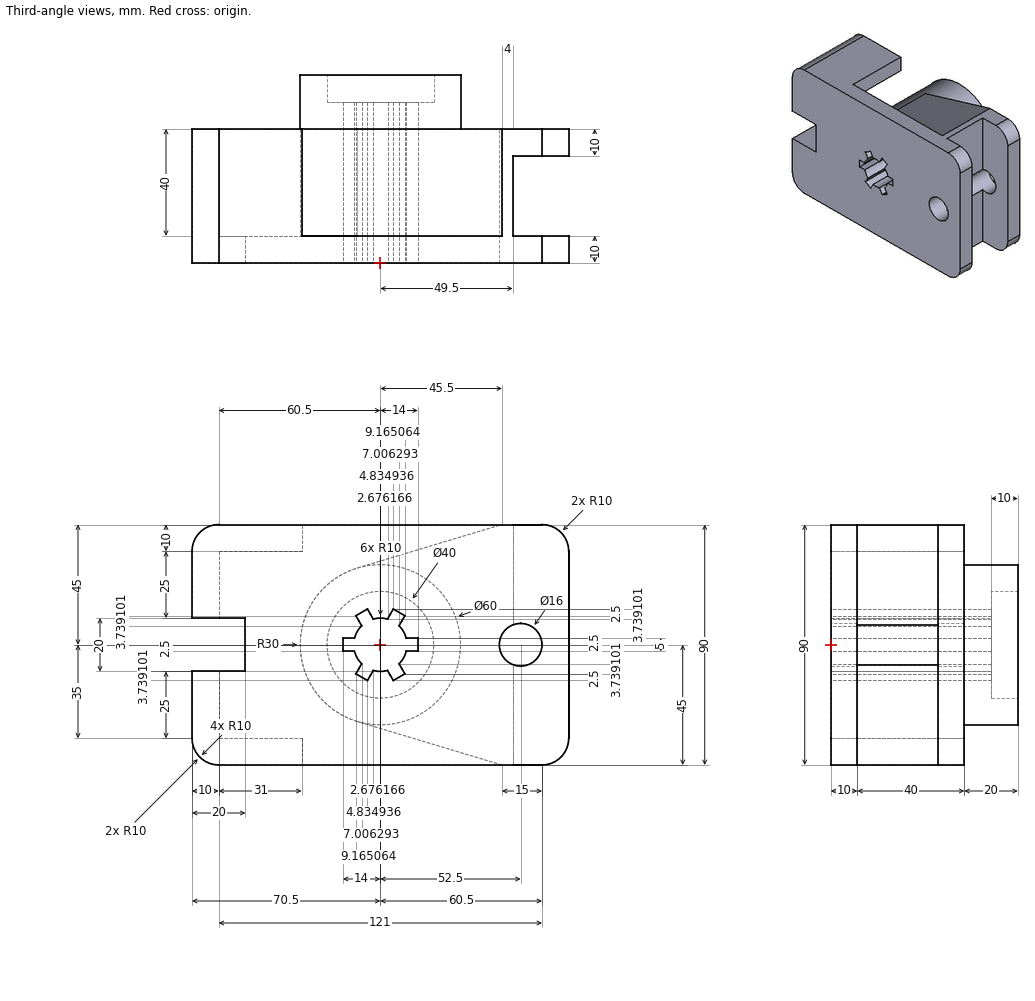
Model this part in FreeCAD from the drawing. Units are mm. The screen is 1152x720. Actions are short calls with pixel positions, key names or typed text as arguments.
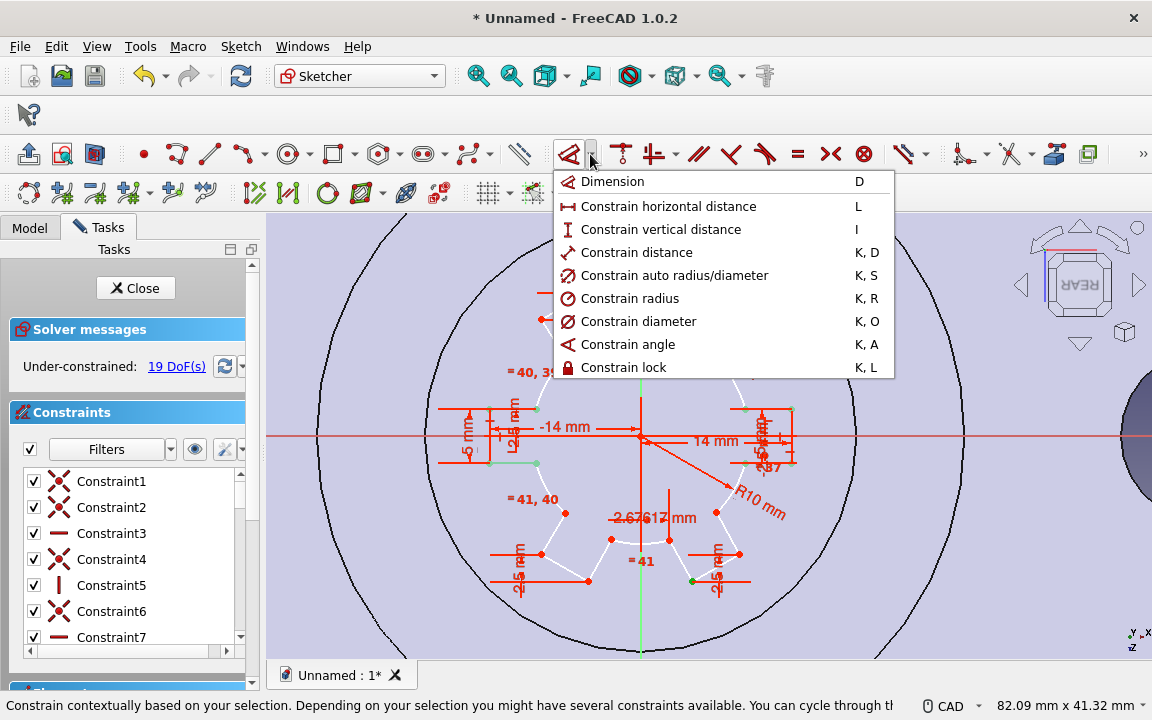
click(724, 206)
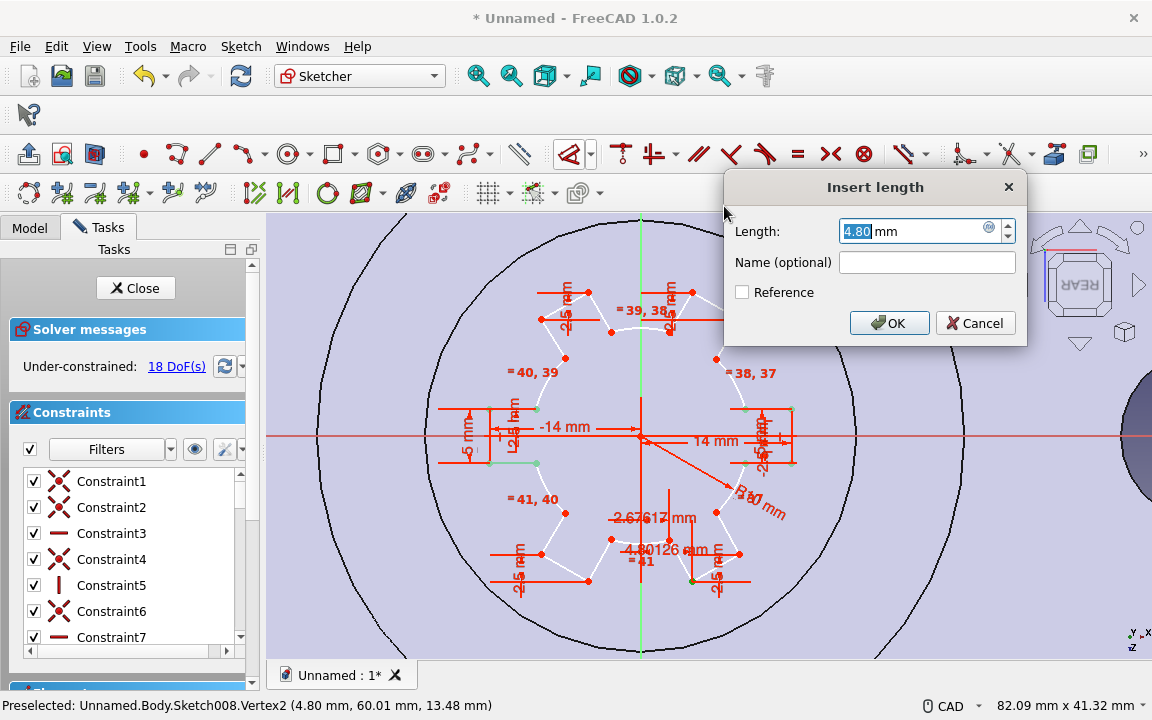
text(4.834936)
key(Return)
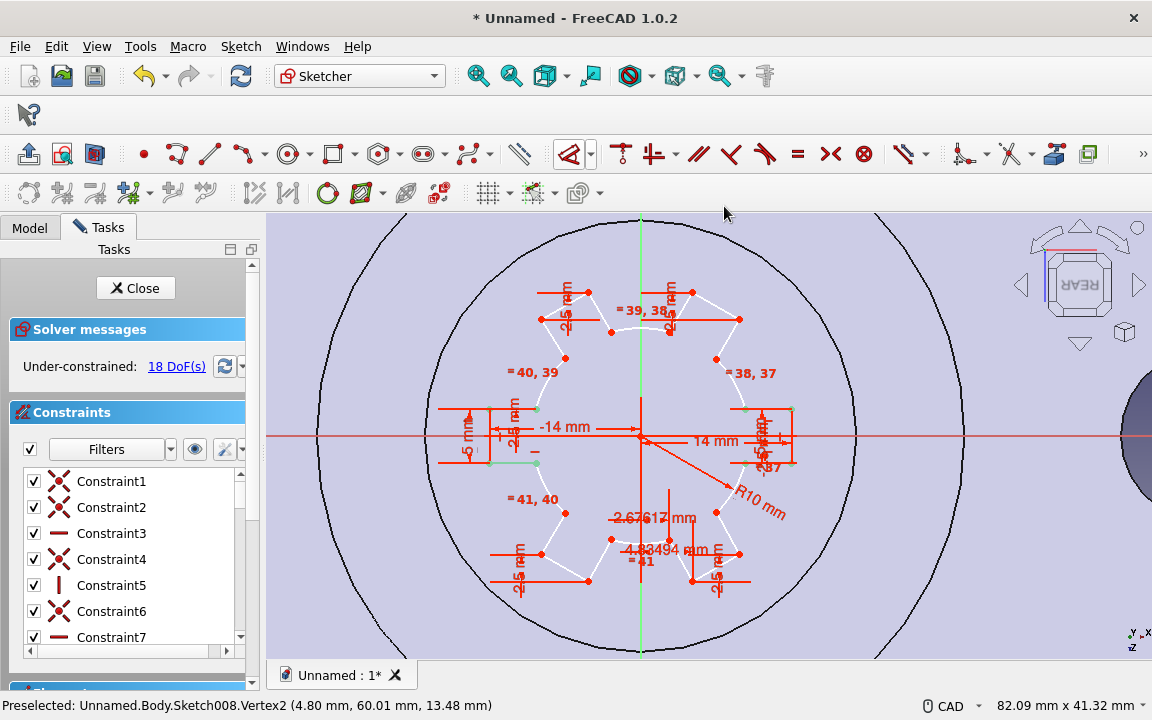
click(739, 555)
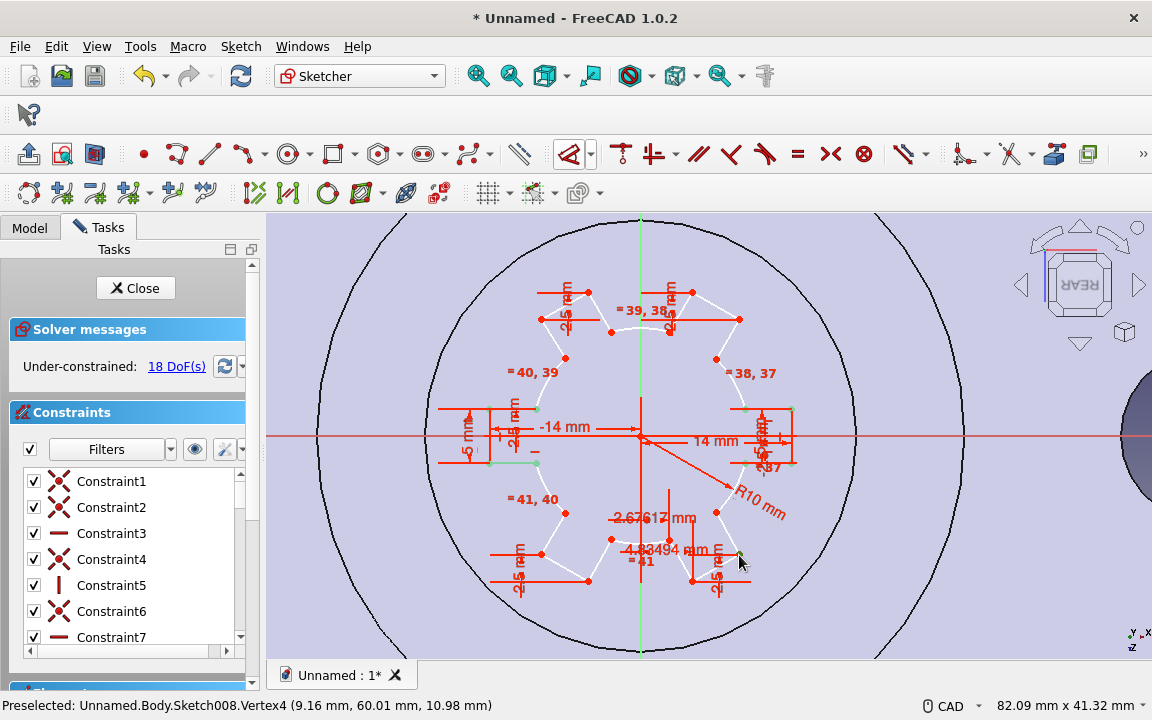
click(590, 154)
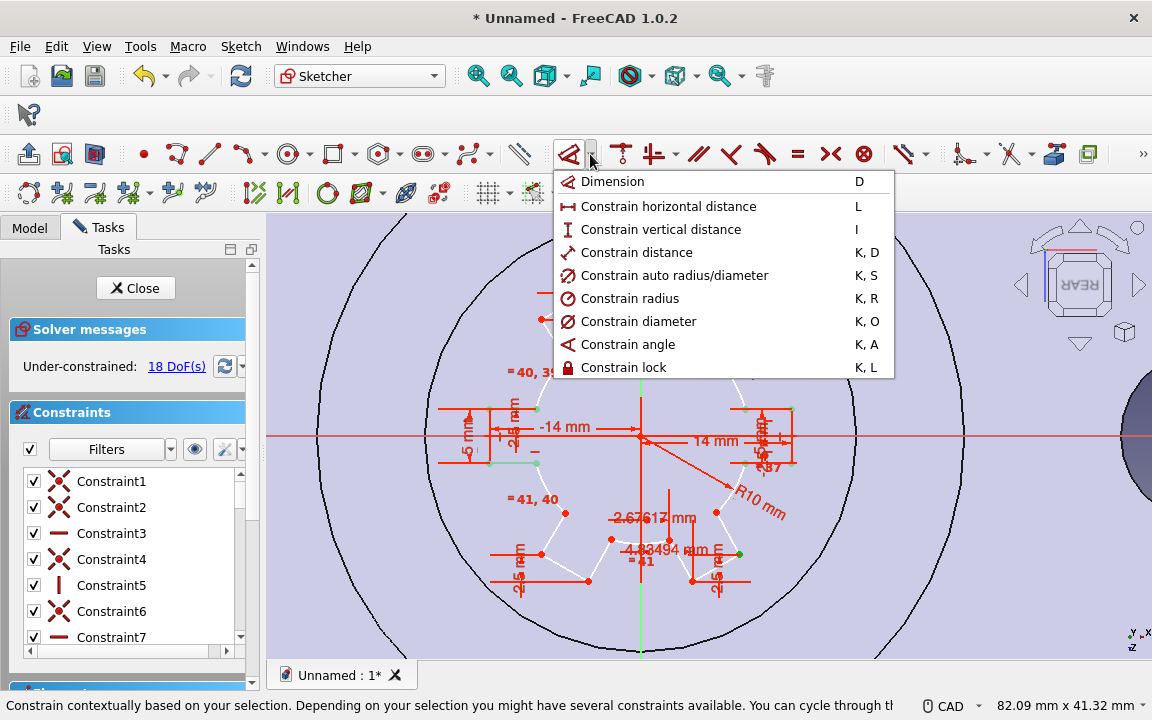
click(724, 206)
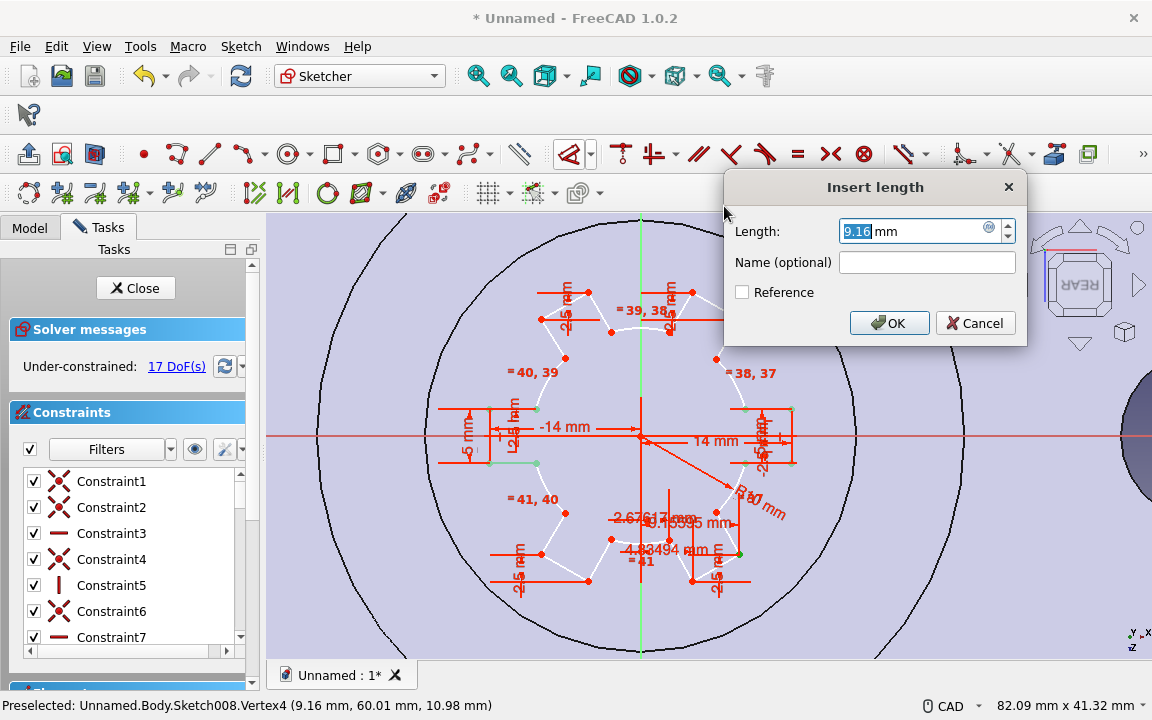
text(9.165064)
key(Return)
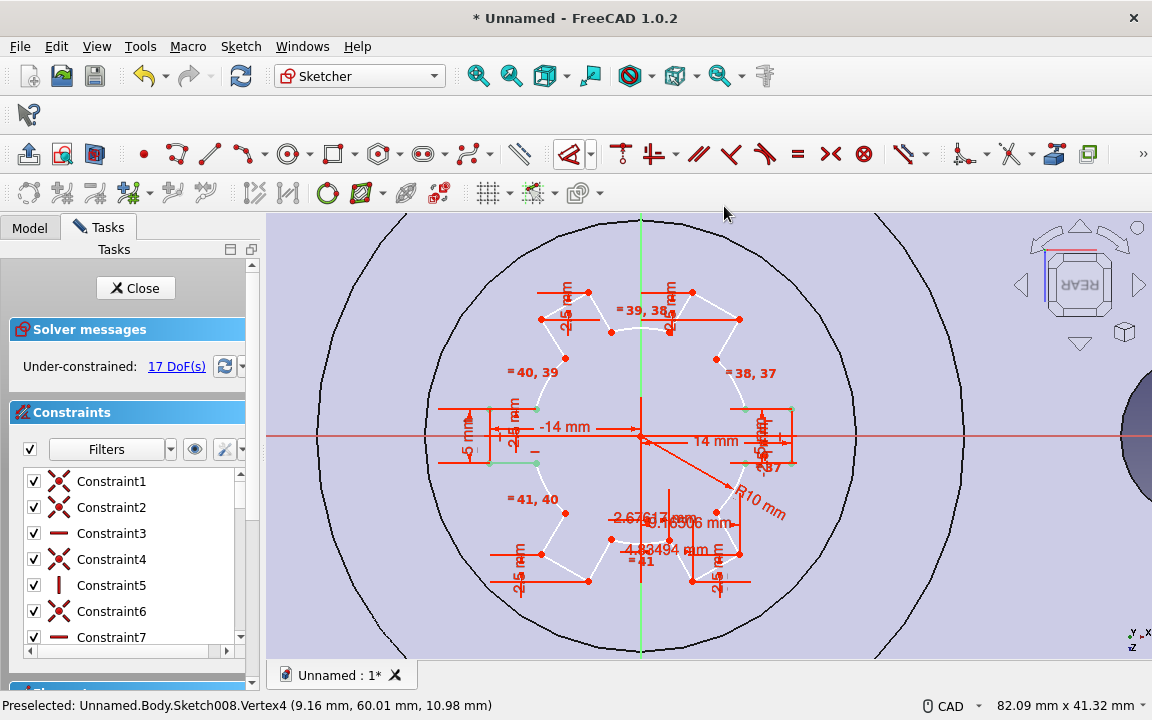
click(717, 513)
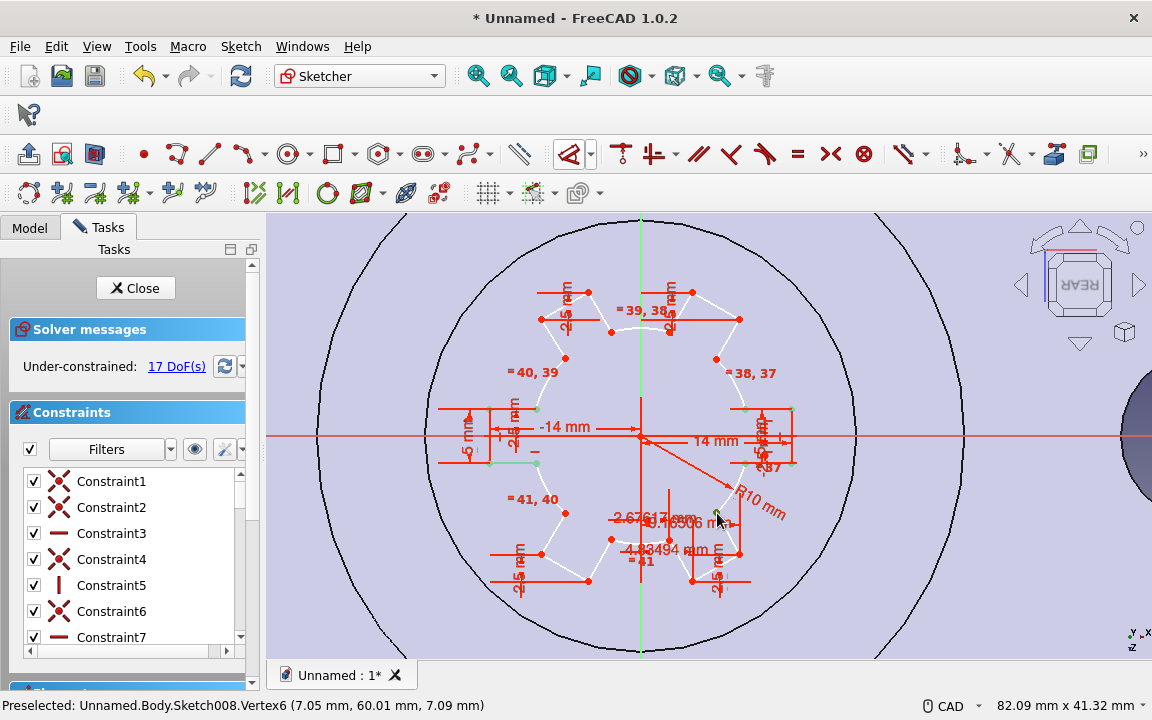
click(590, 154)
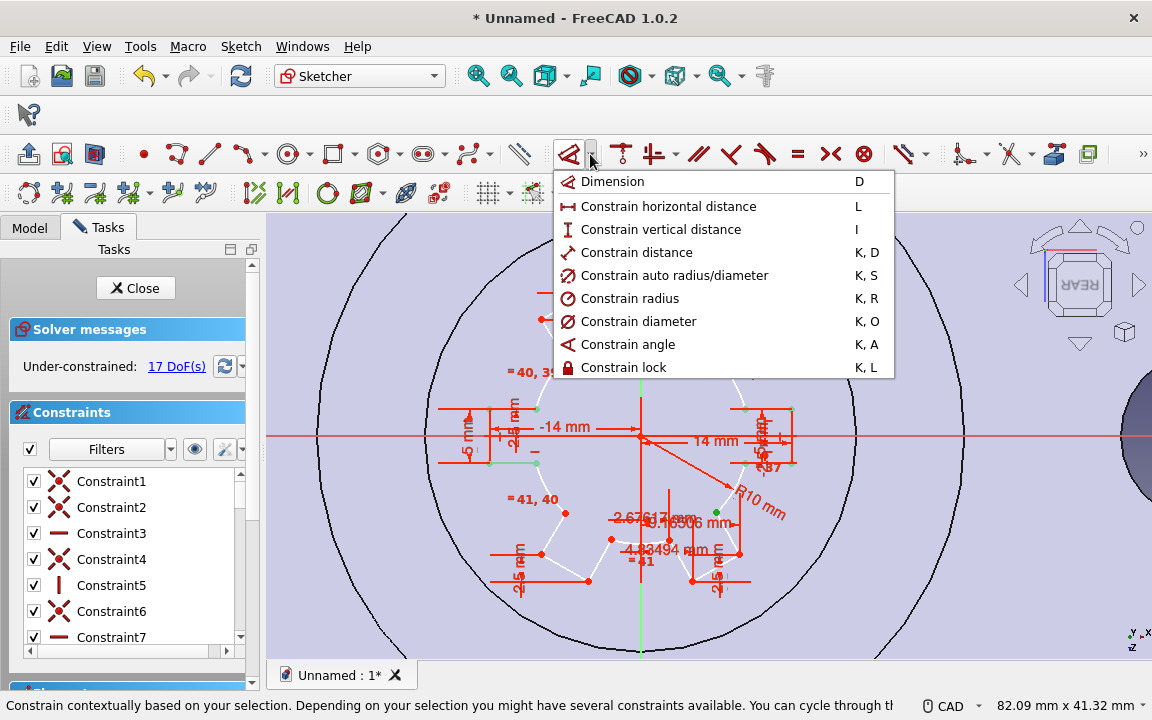
click(724, 206)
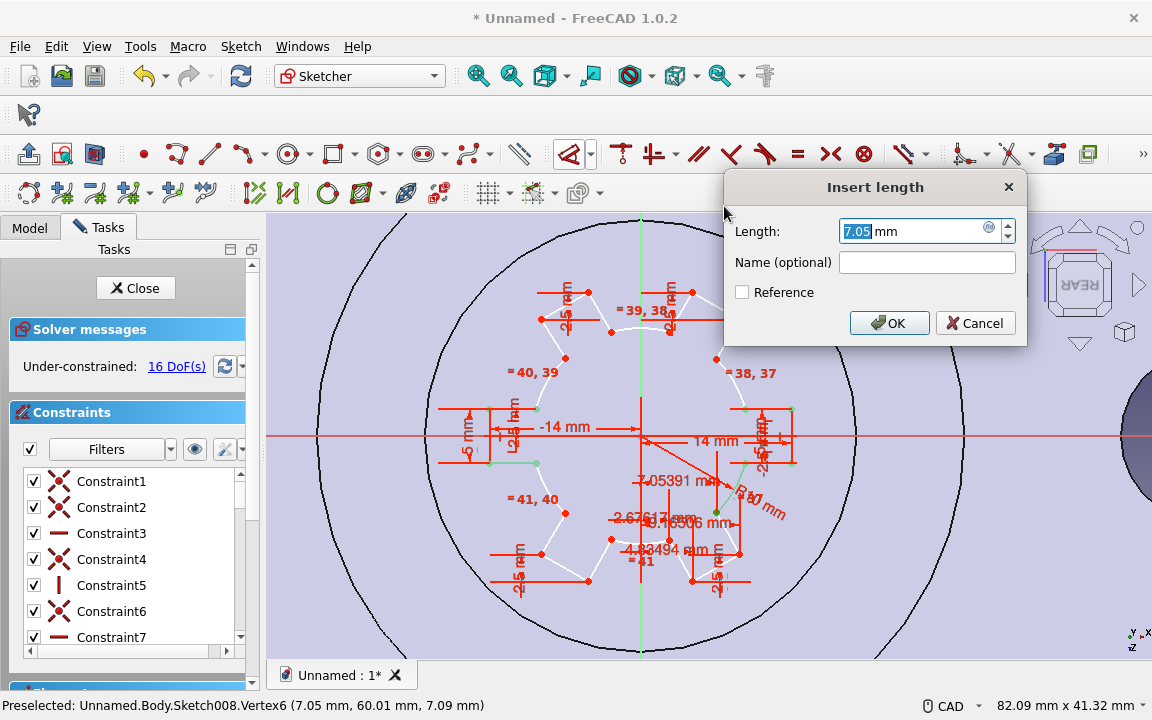
text(7.006293)
key(Return)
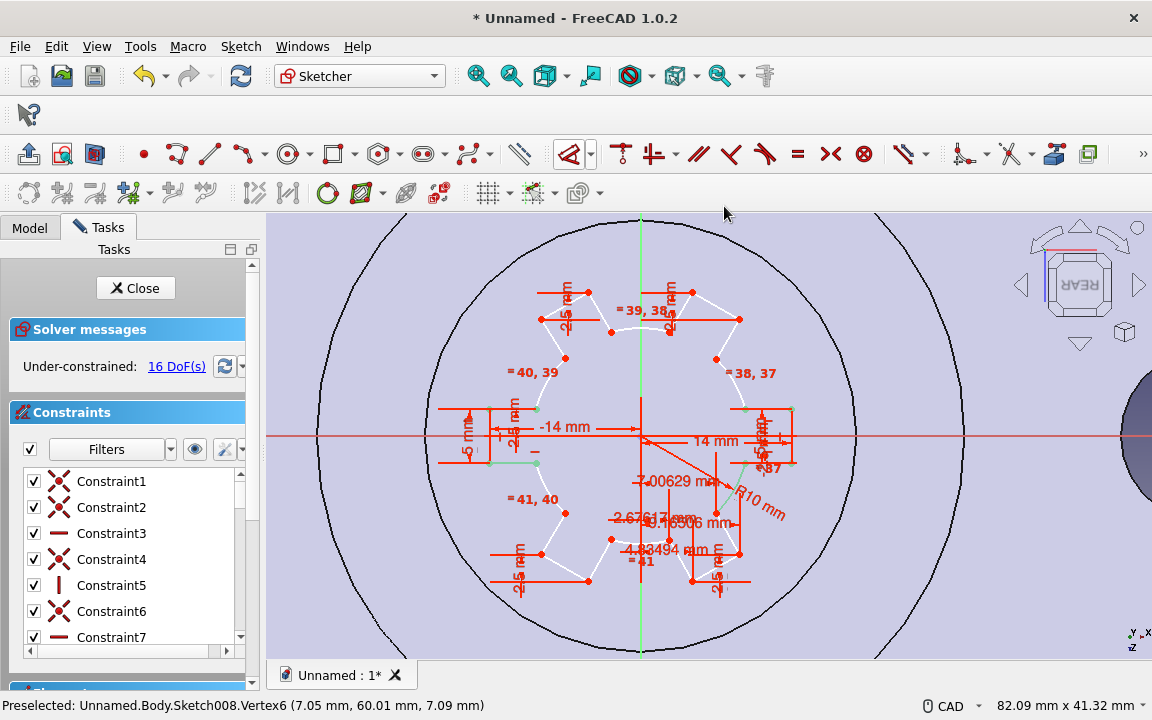
click(717, 359)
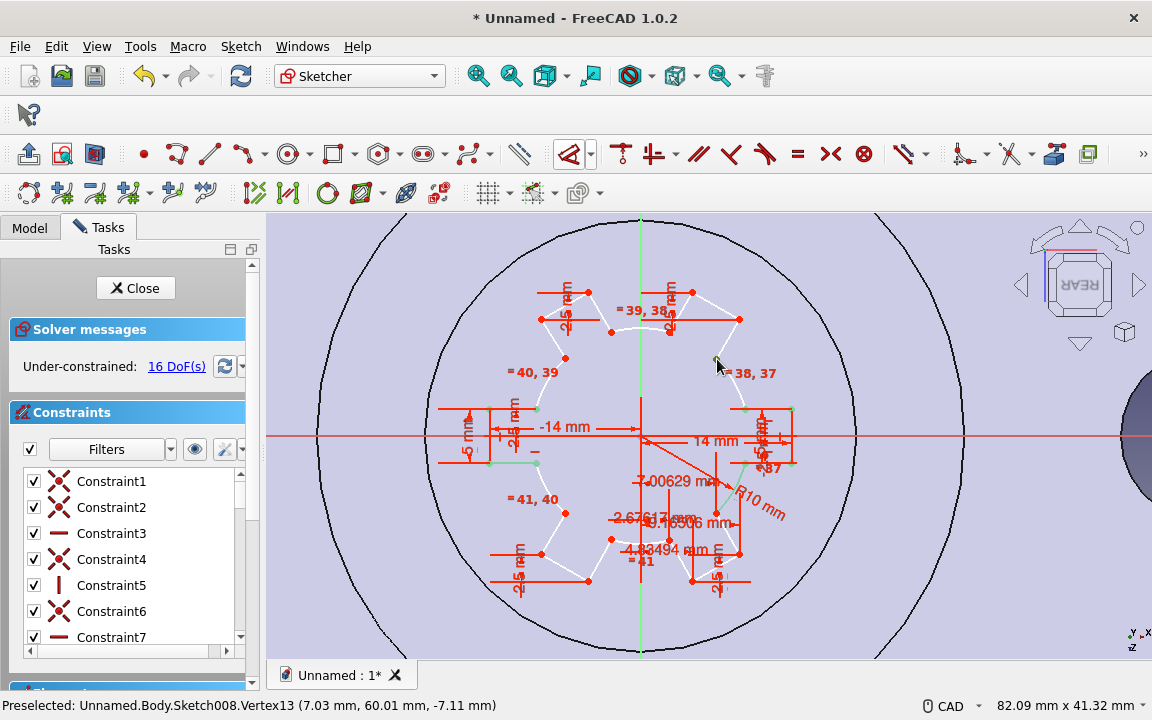
click(590, 154)